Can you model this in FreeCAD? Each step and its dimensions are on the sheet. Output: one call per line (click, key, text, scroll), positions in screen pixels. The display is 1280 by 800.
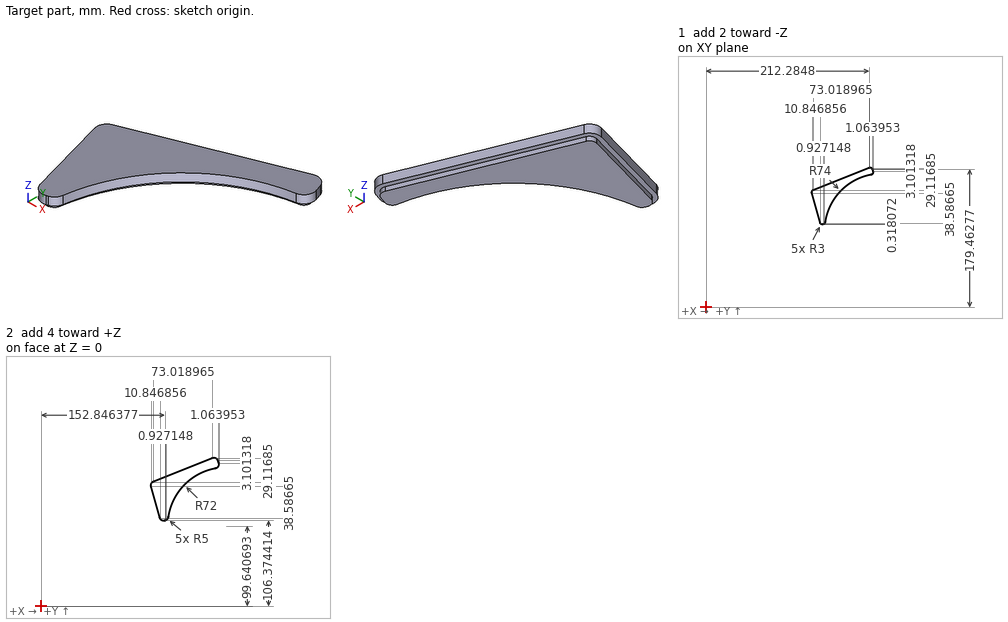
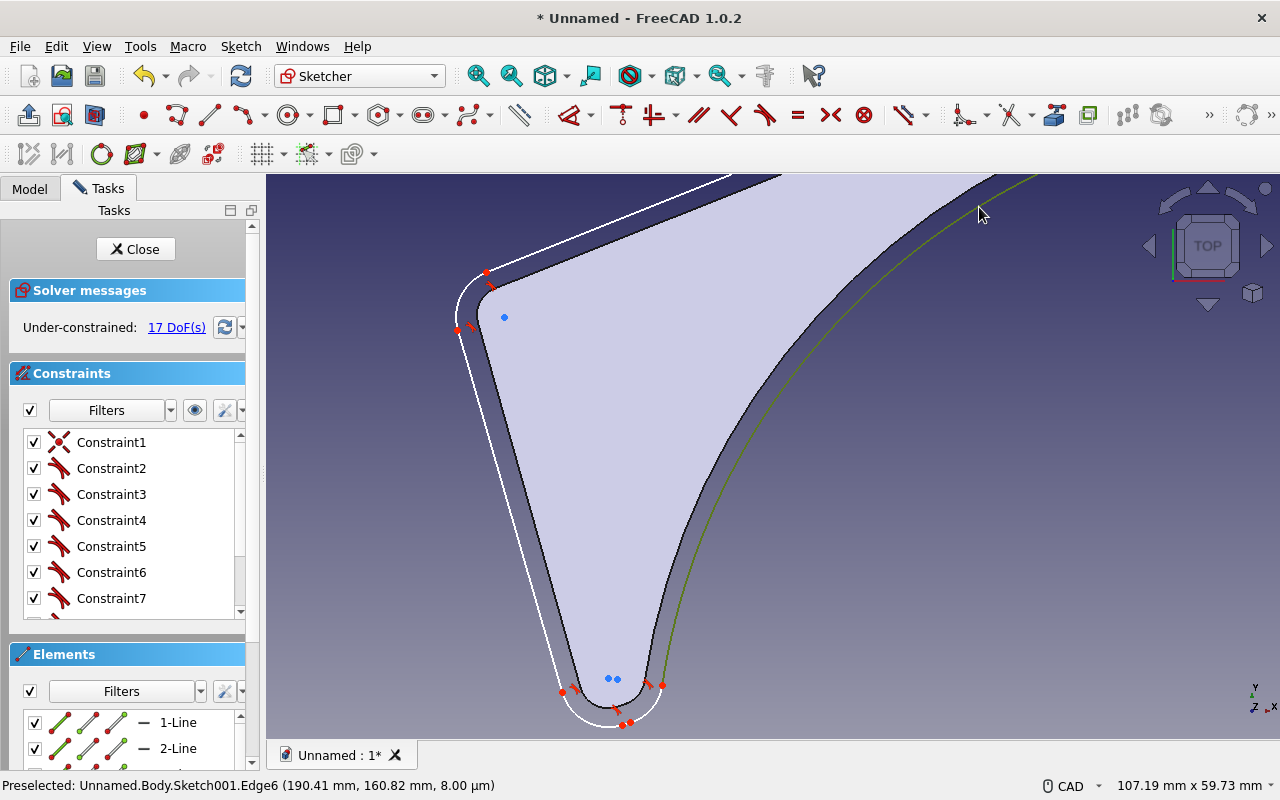
scroll(582, 535, down, 4)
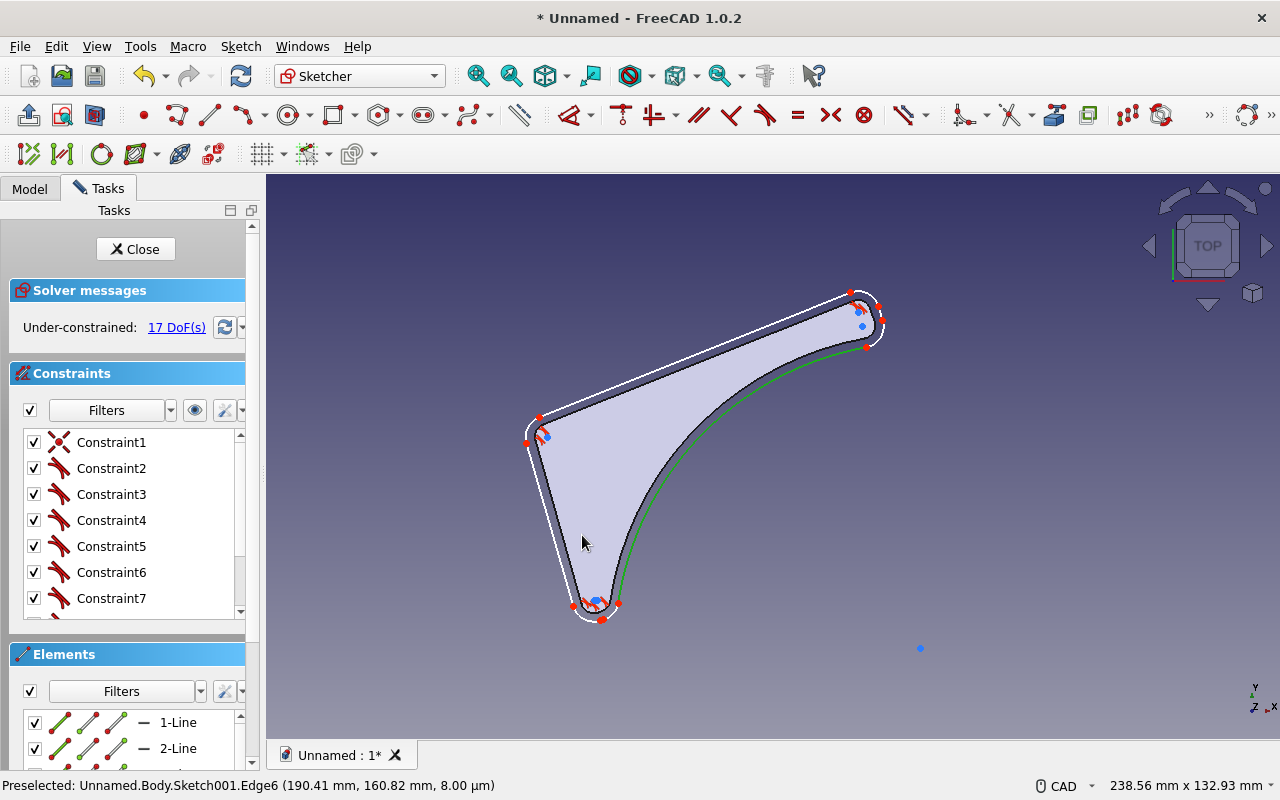
scroll(876, 343, up, 2)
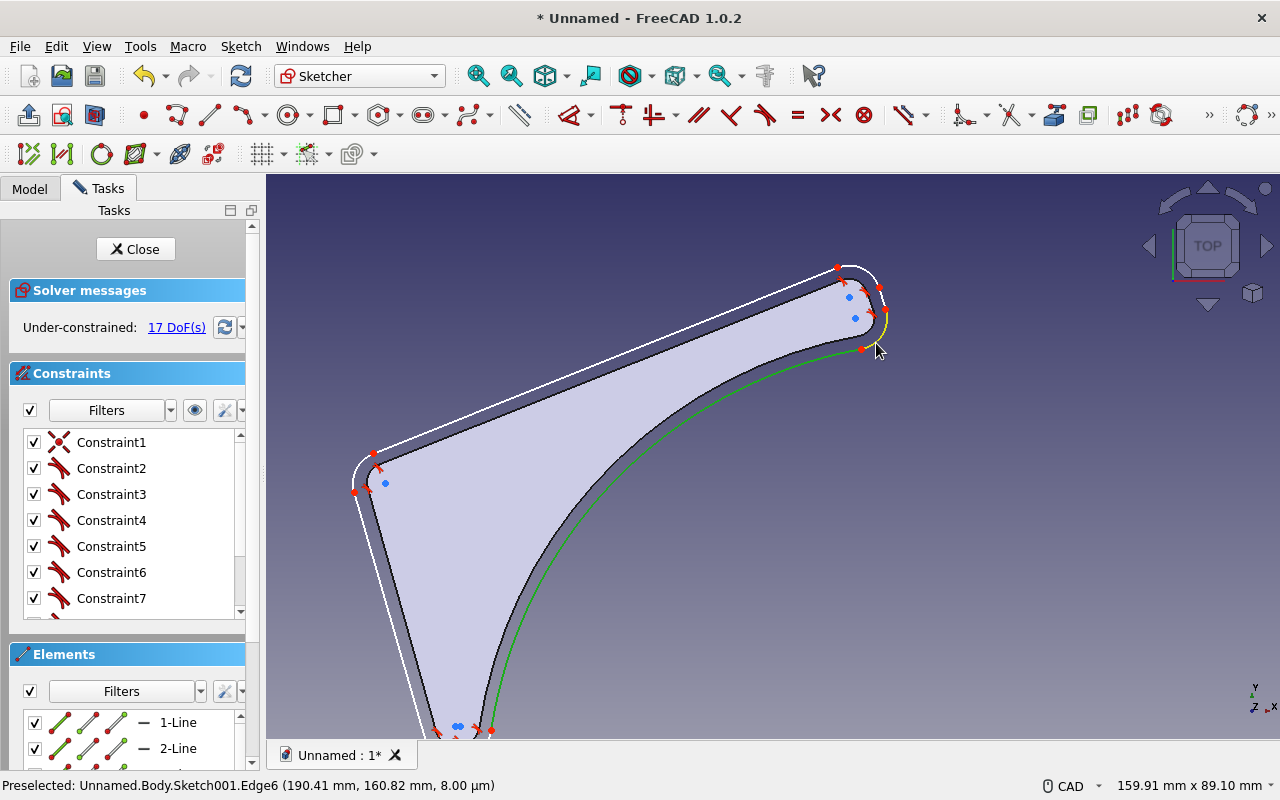
click(876, 343)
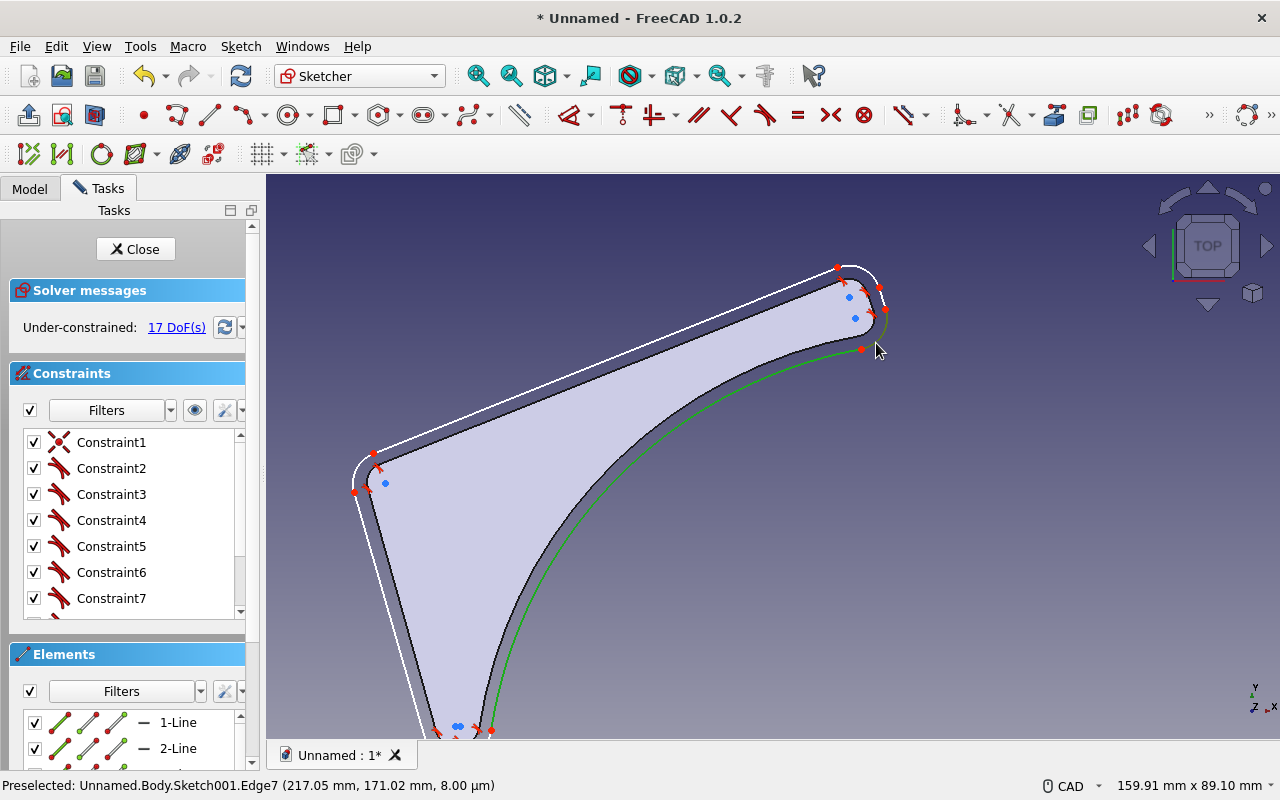
click(765, 116)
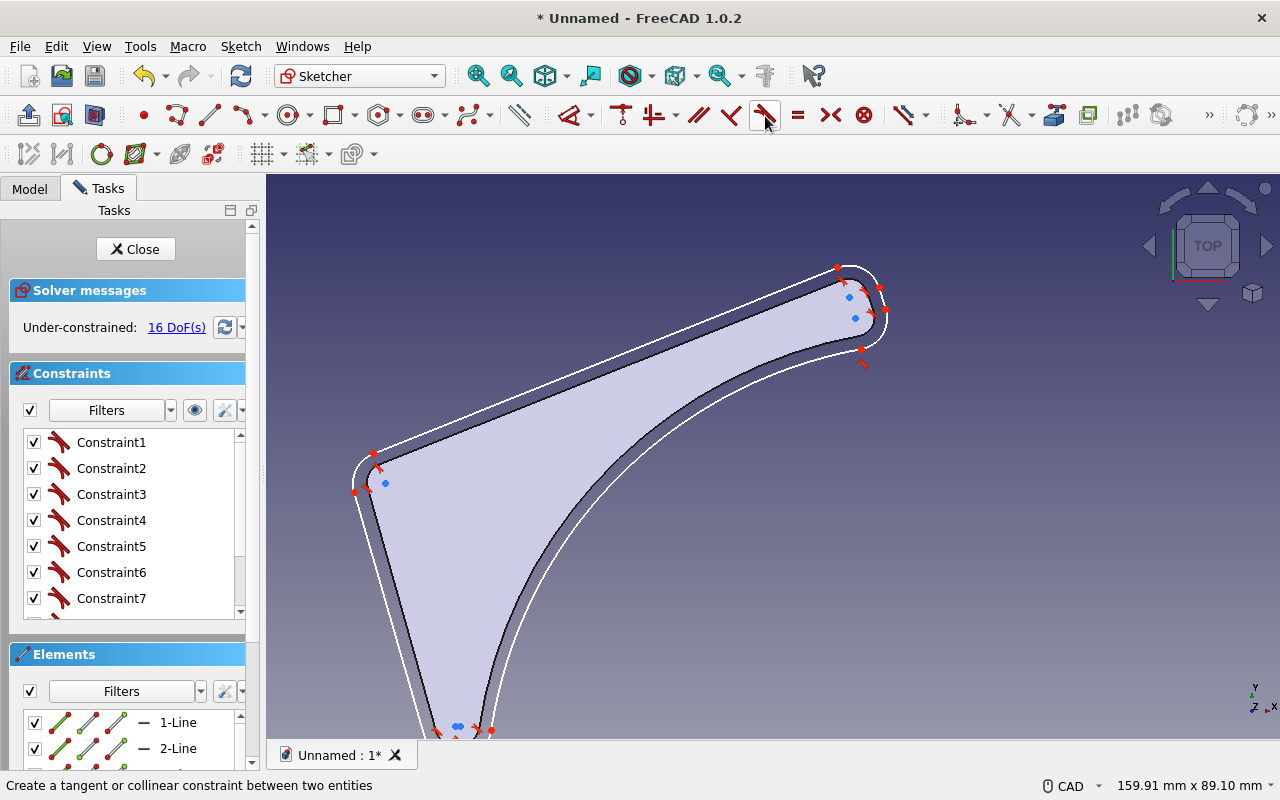
scroll(875, 342, down, 2)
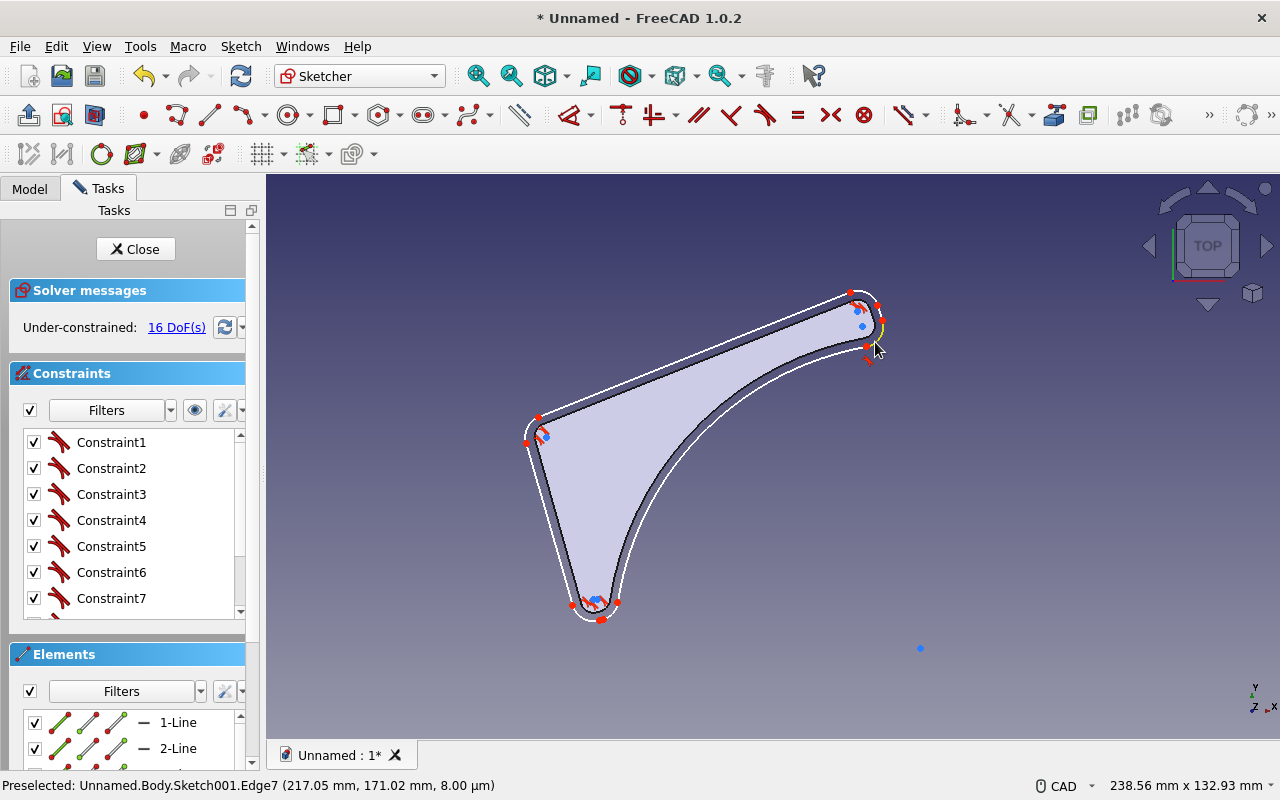
scroll(610, 616, up, 4)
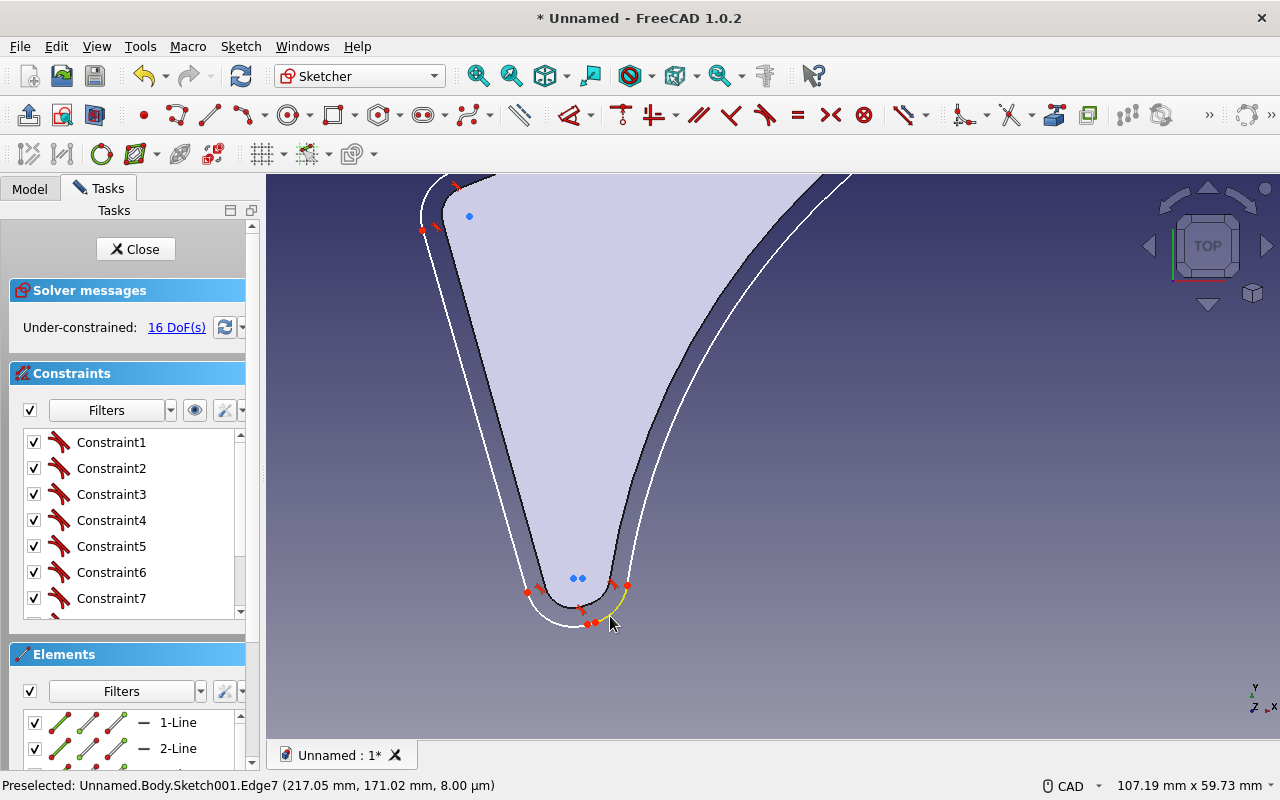
click(609, 616)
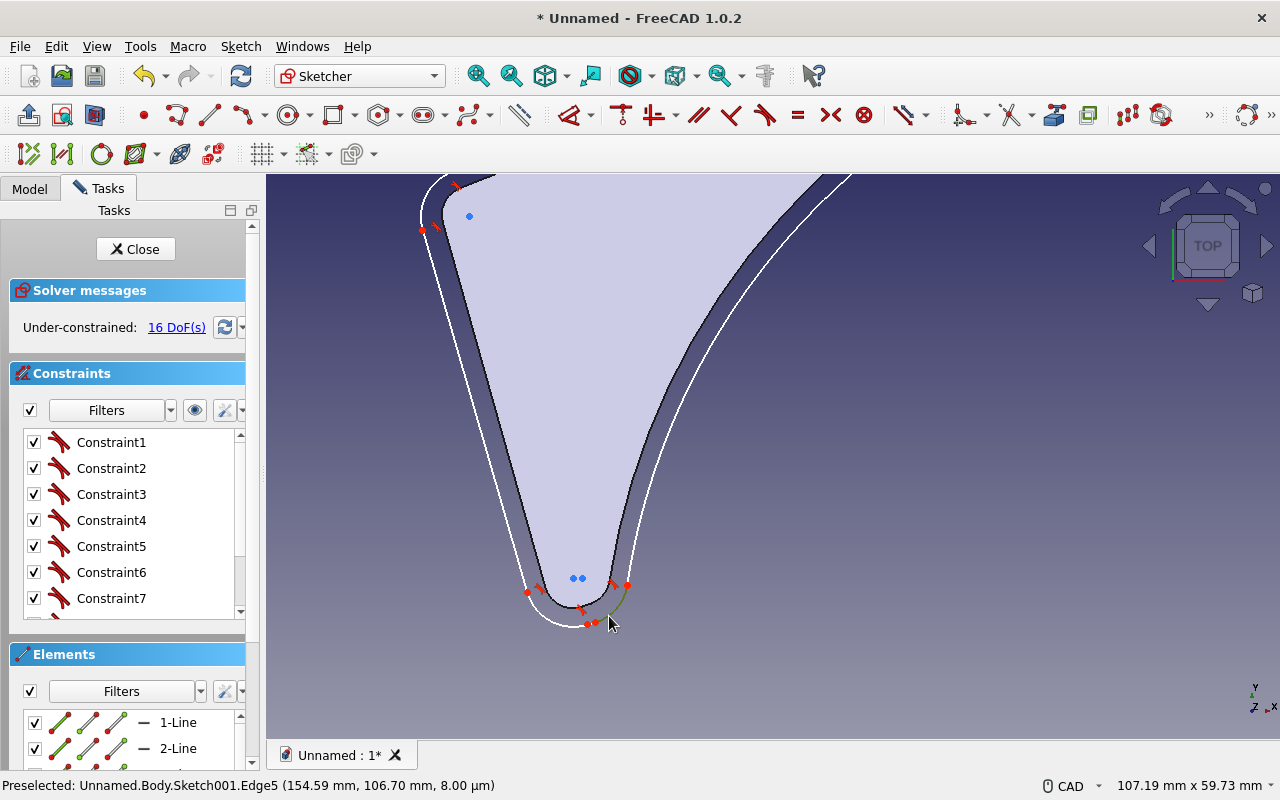
scroll(610, 617, down, 4)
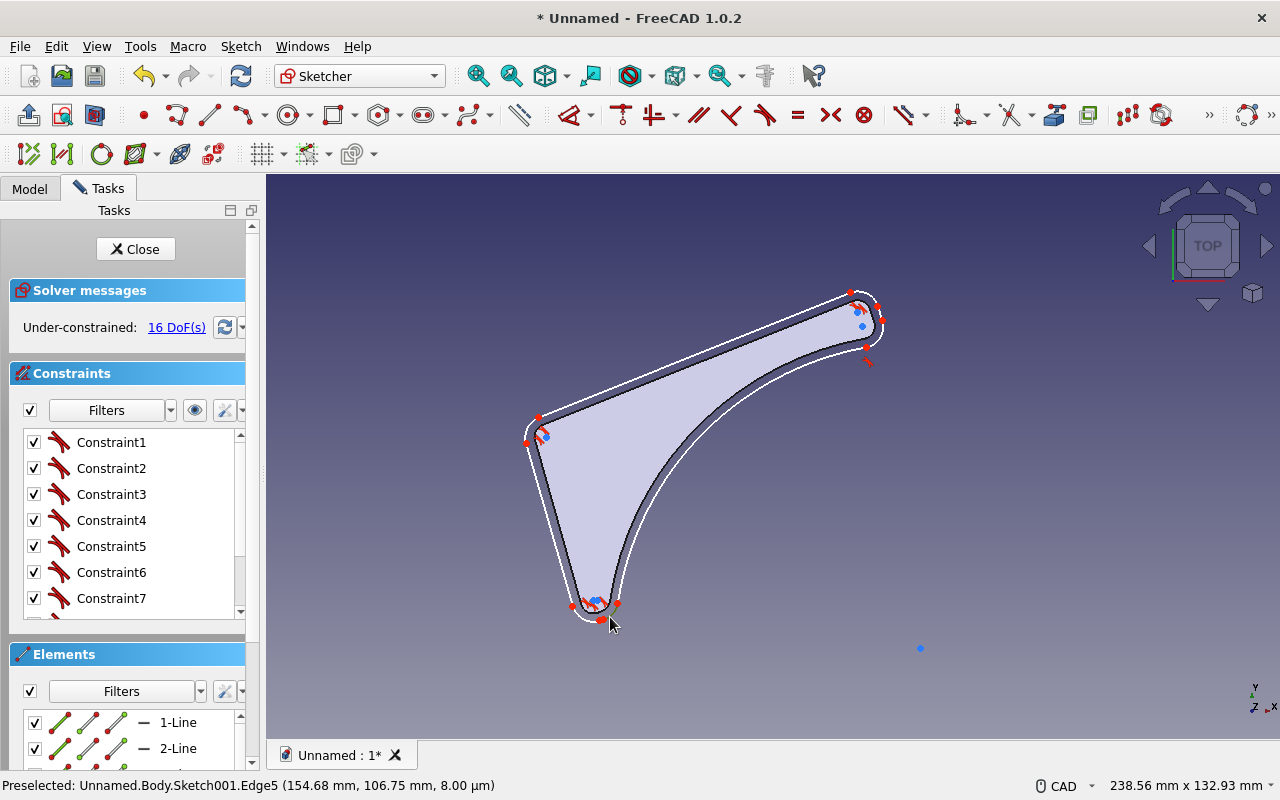
scroll(876, 343, up, 2)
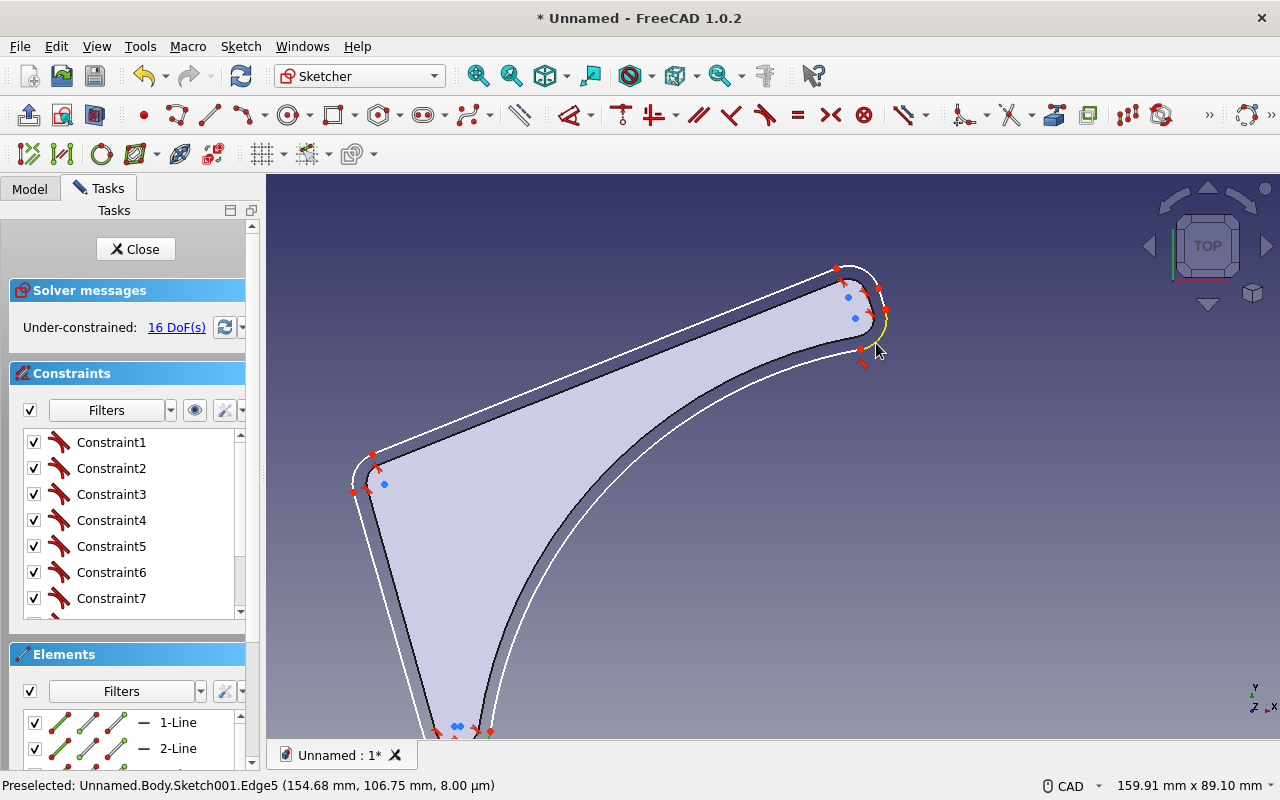
click(875, 343)